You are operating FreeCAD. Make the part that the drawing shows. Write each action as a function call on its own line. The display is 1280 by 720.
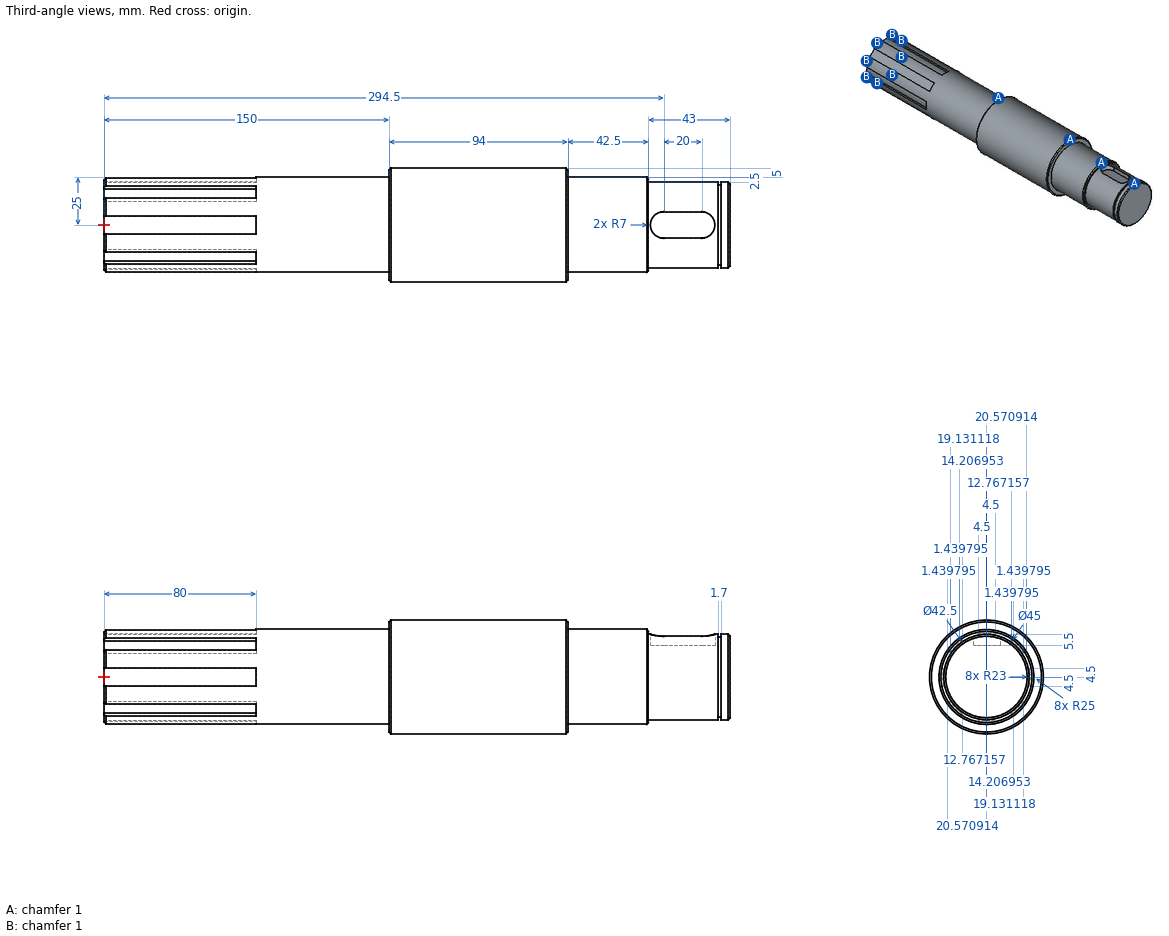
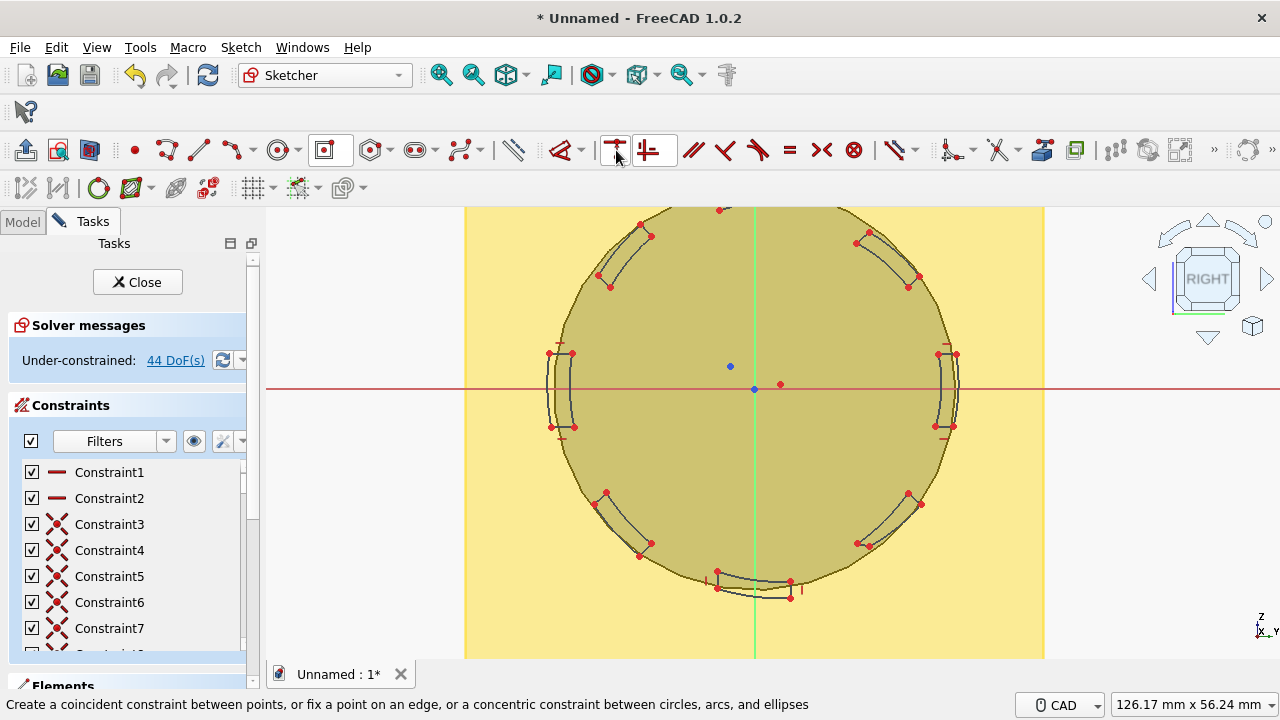
click(940, 405)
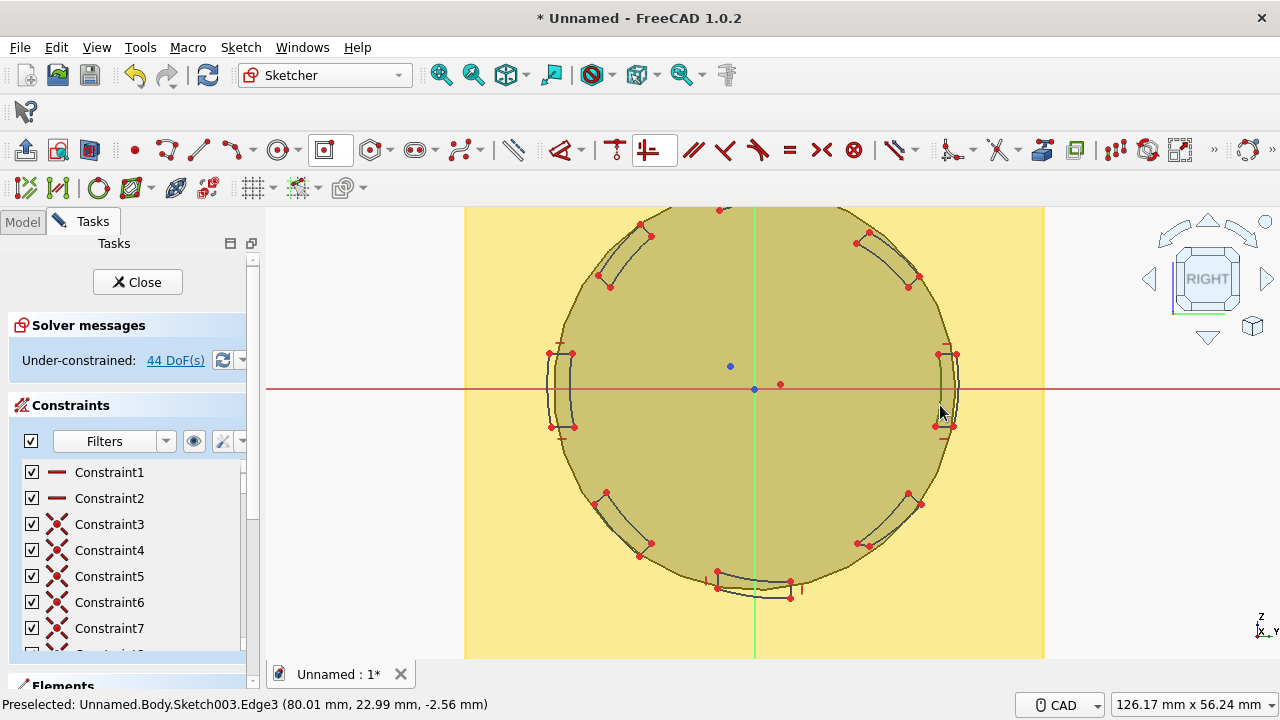
scroll(874, 531, up, 2)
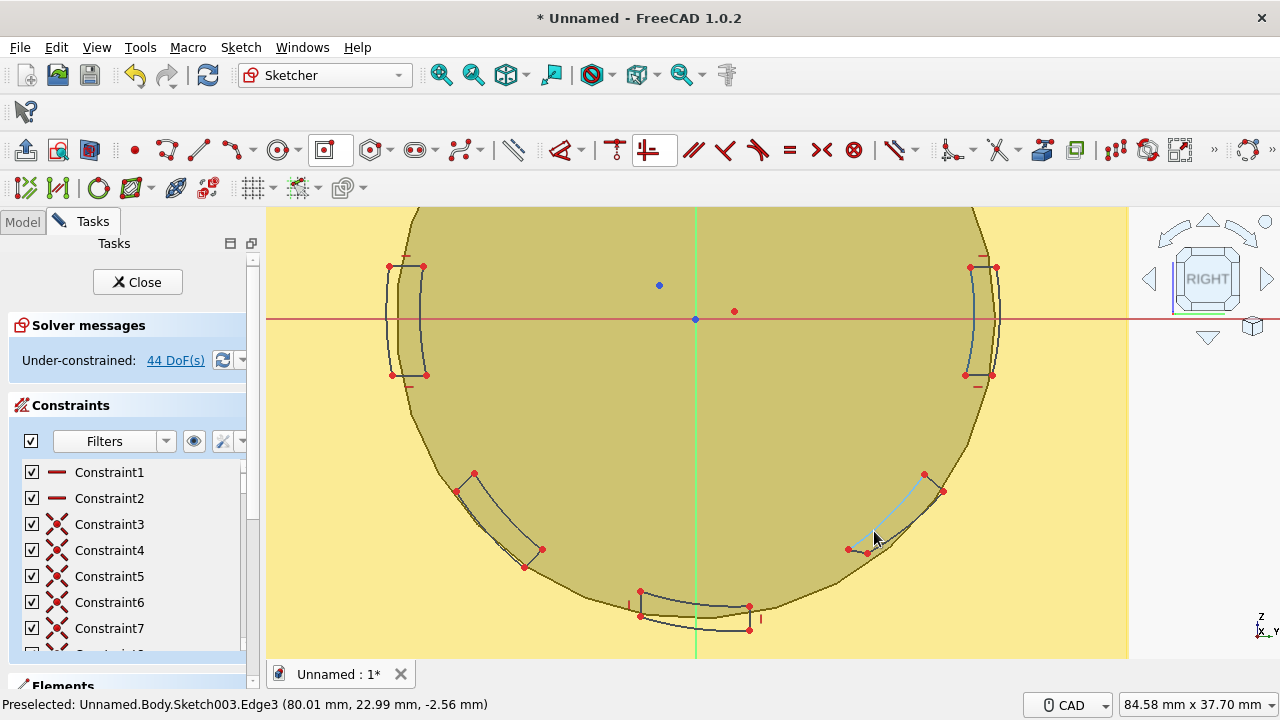
click(874, 530)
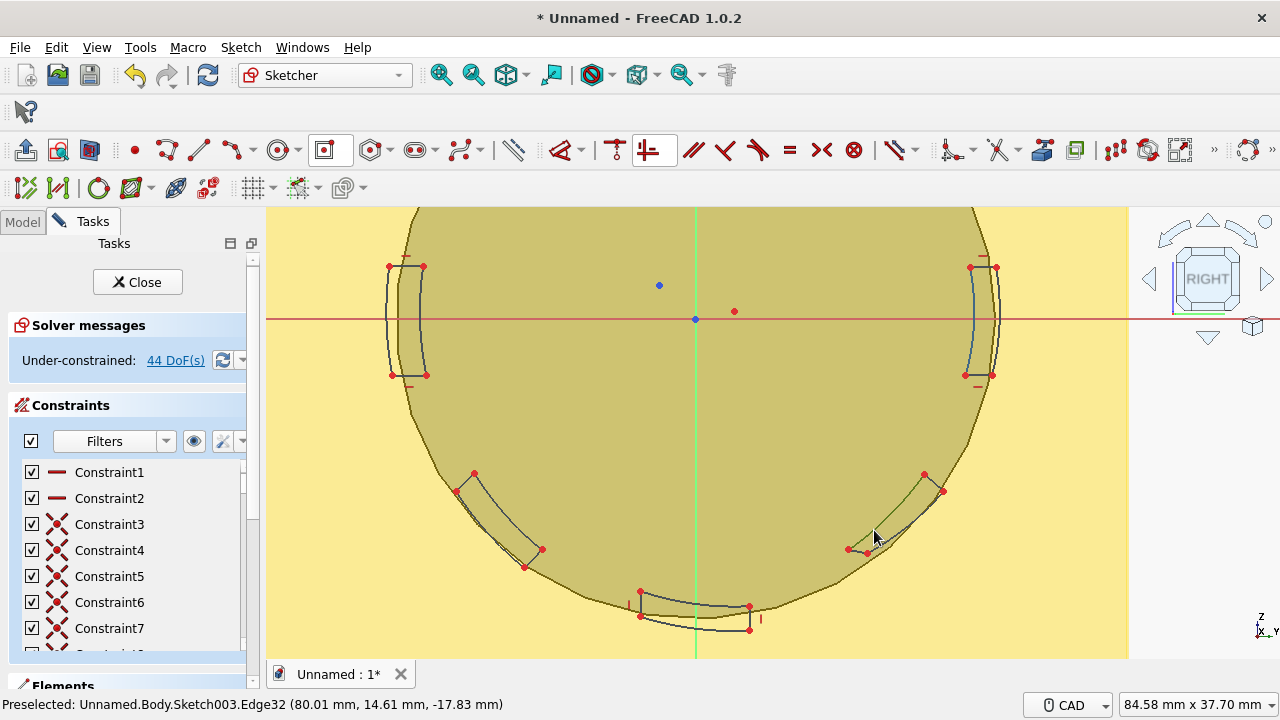
click(616, 150)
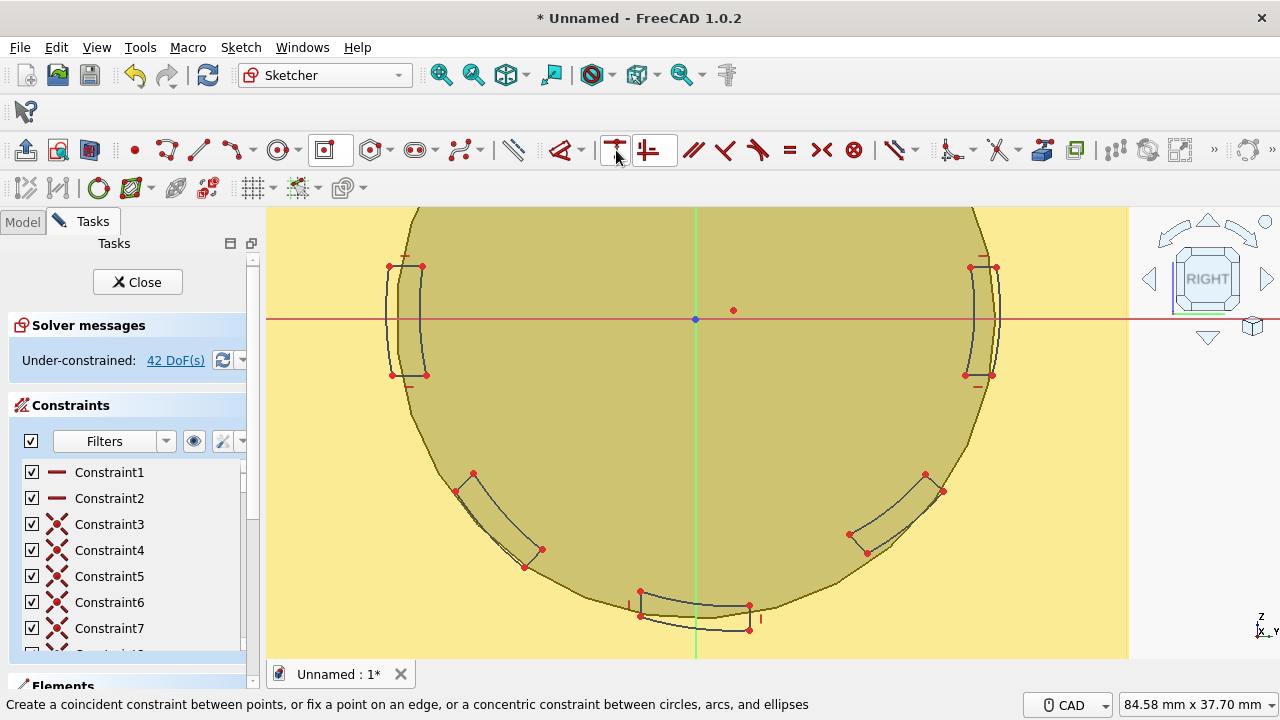
drag(686, 301, 744, 329)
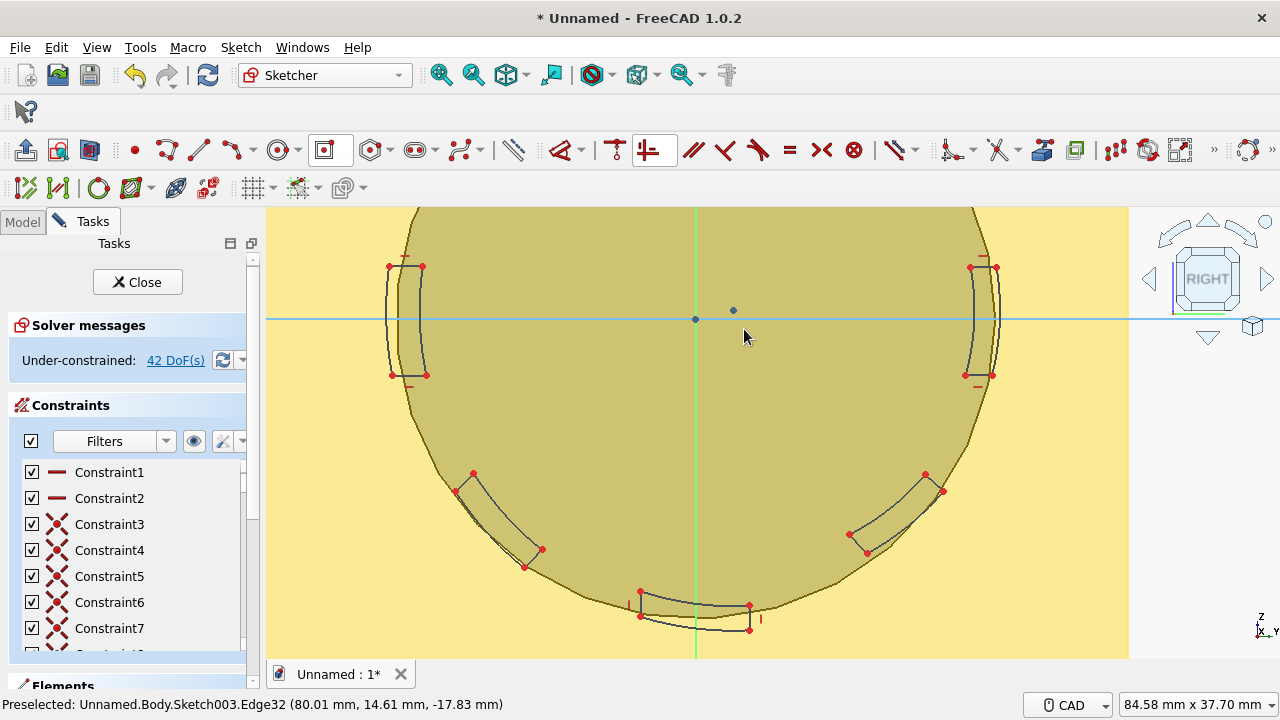
click(616, 150)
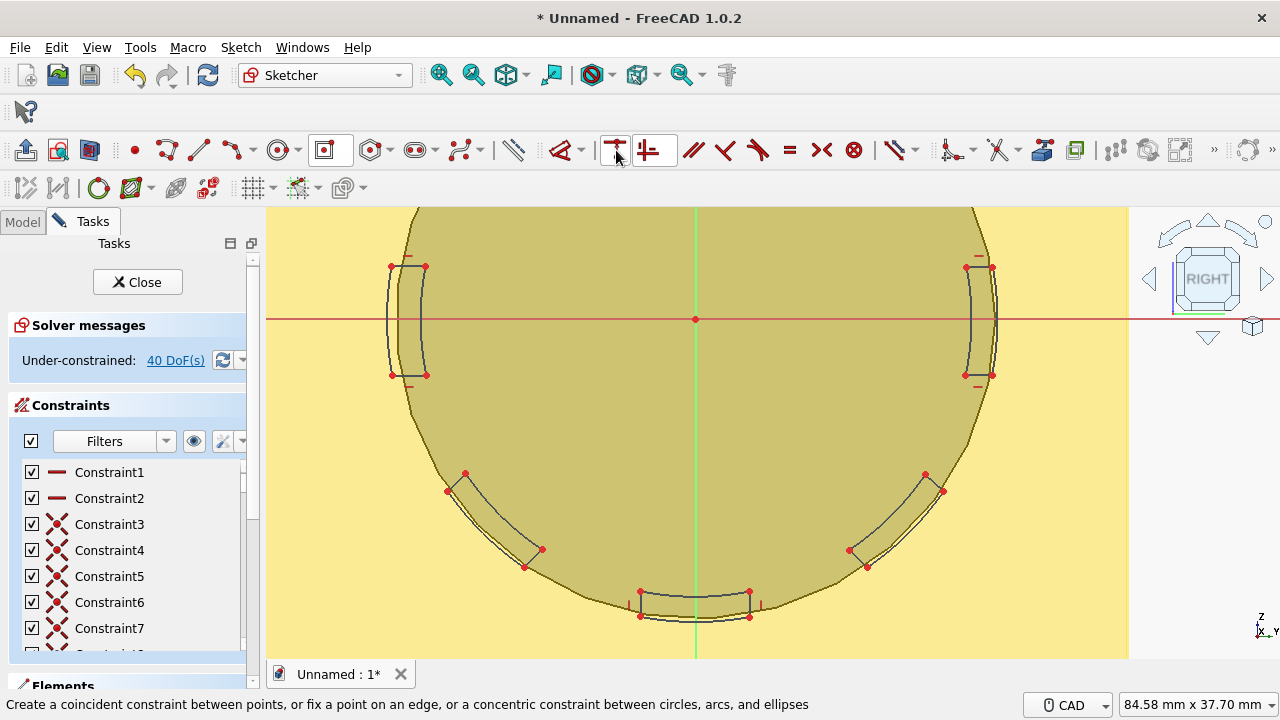
click(996, 343)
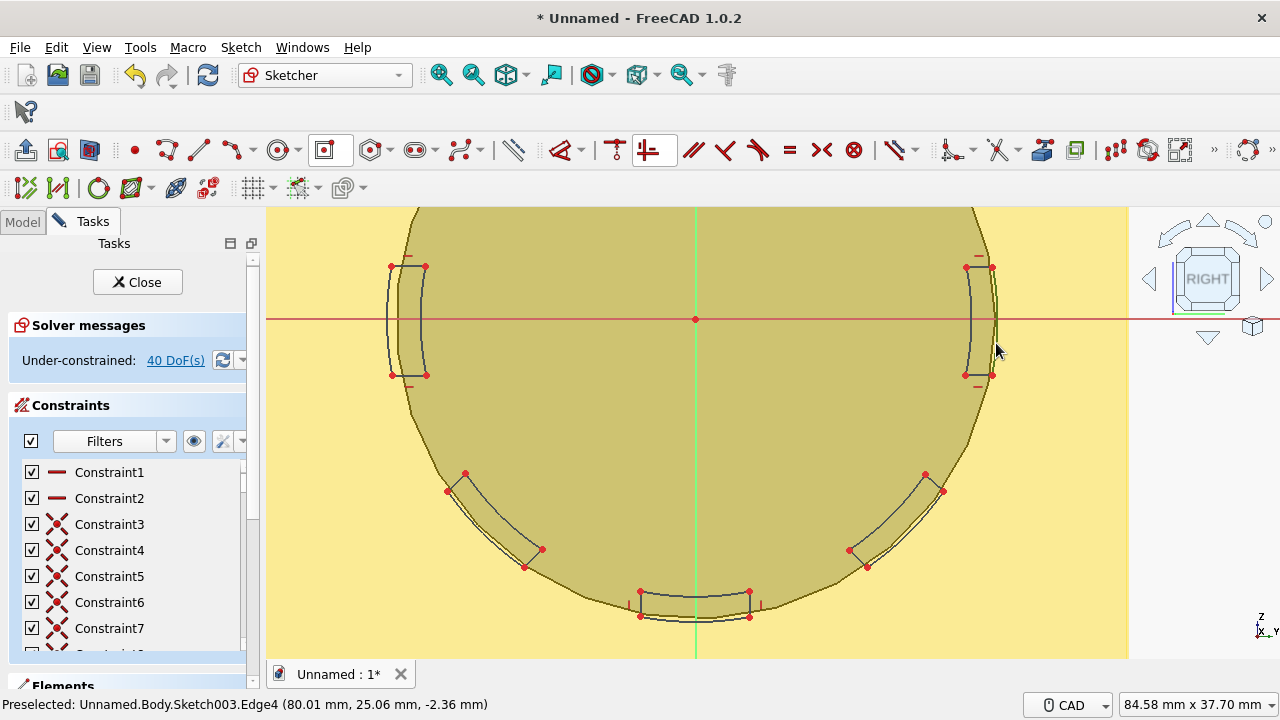
scroll(712, 526, down, 4)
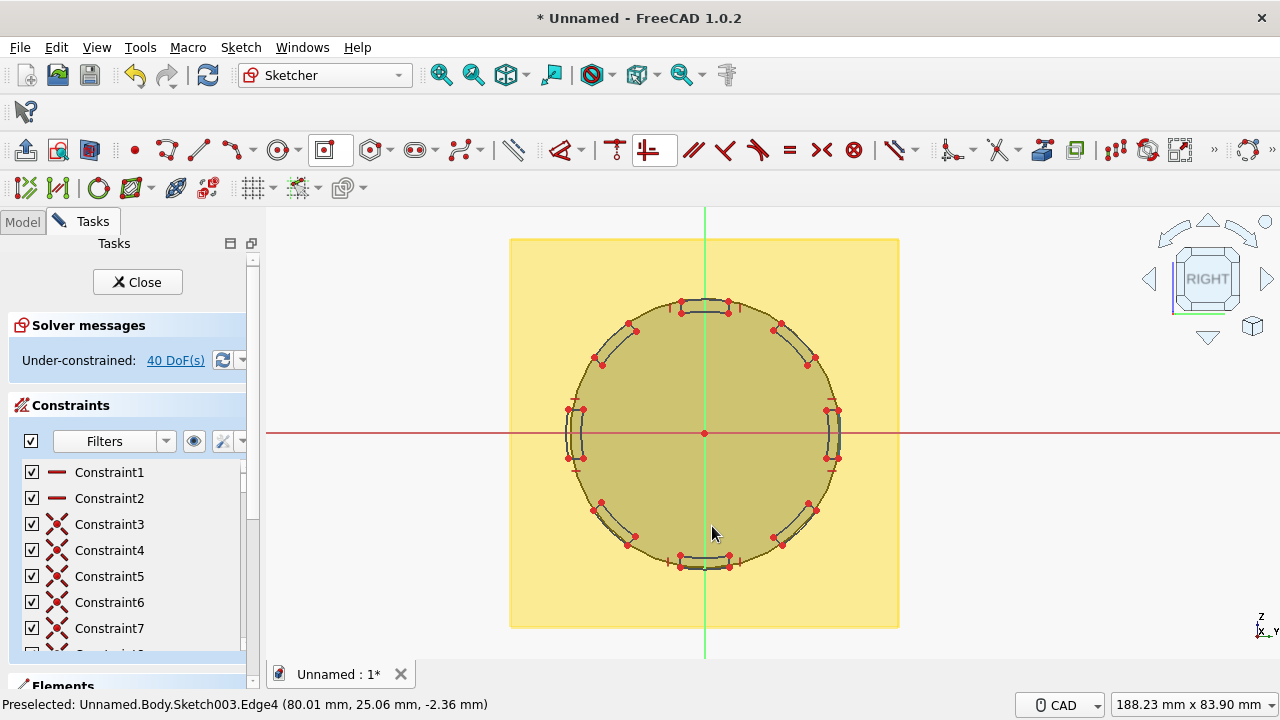
scroll(807, 346, up, 2)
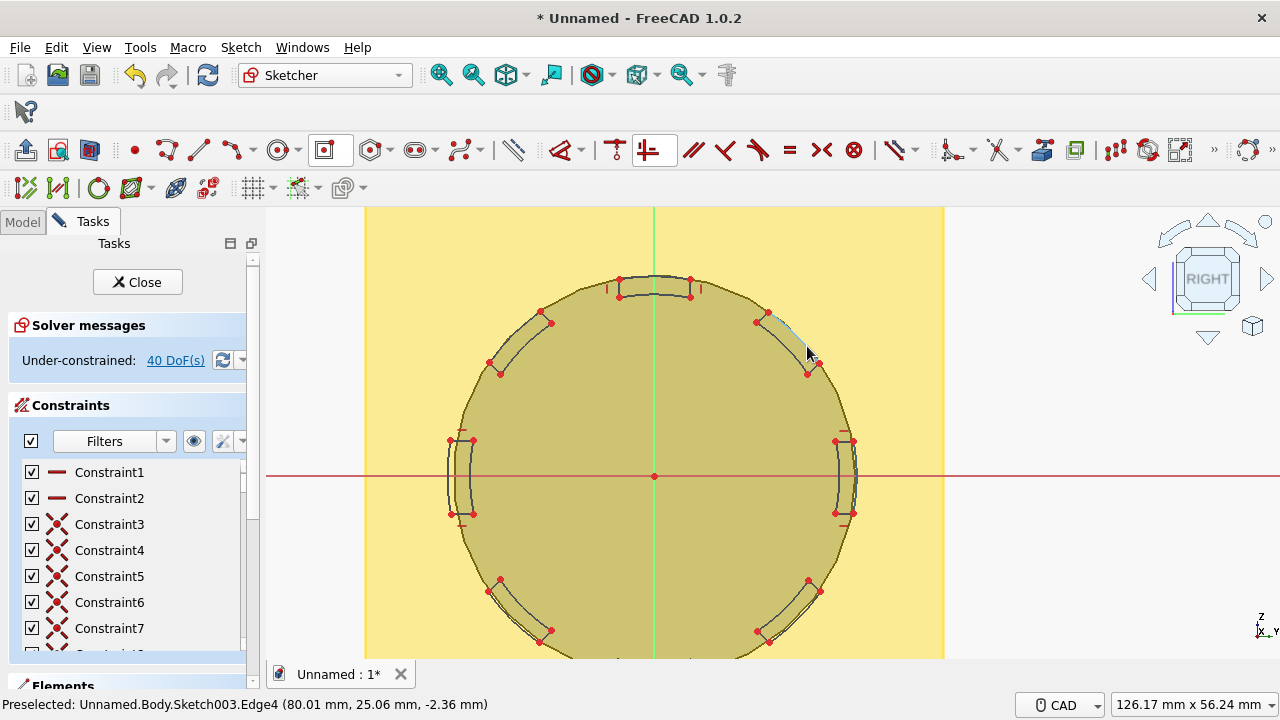
click(806, 346)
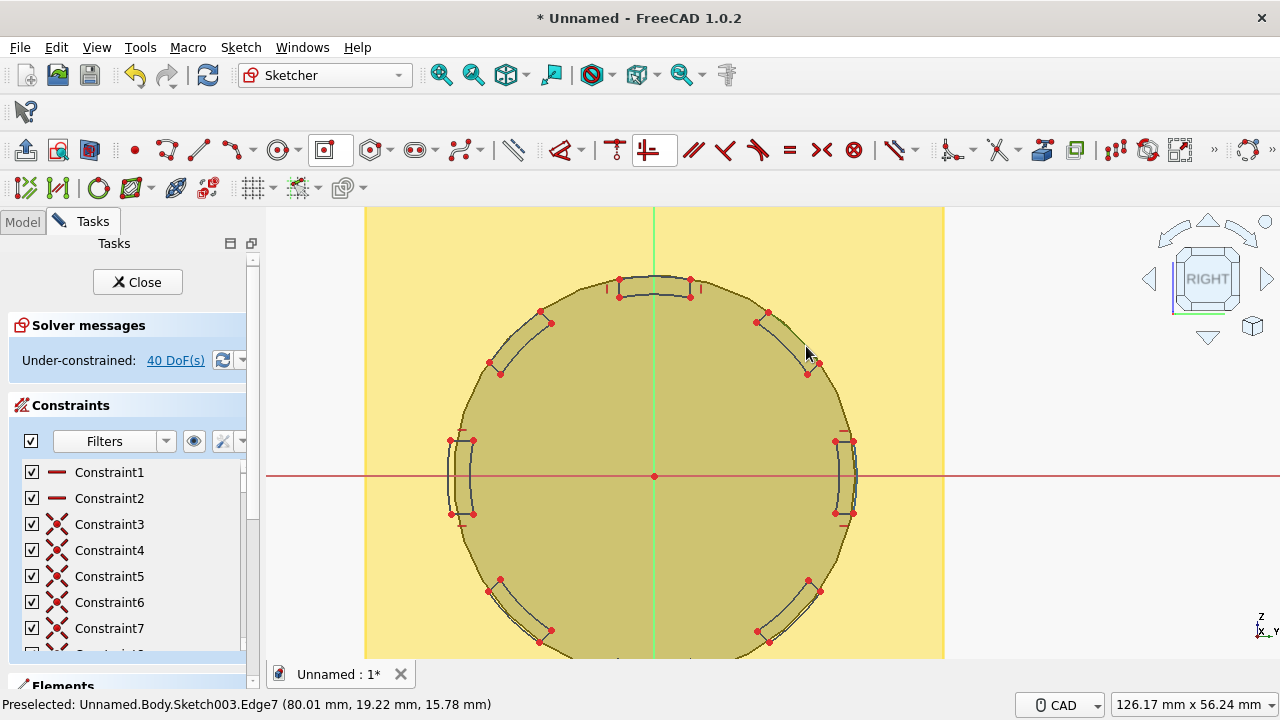
click(669, 277)